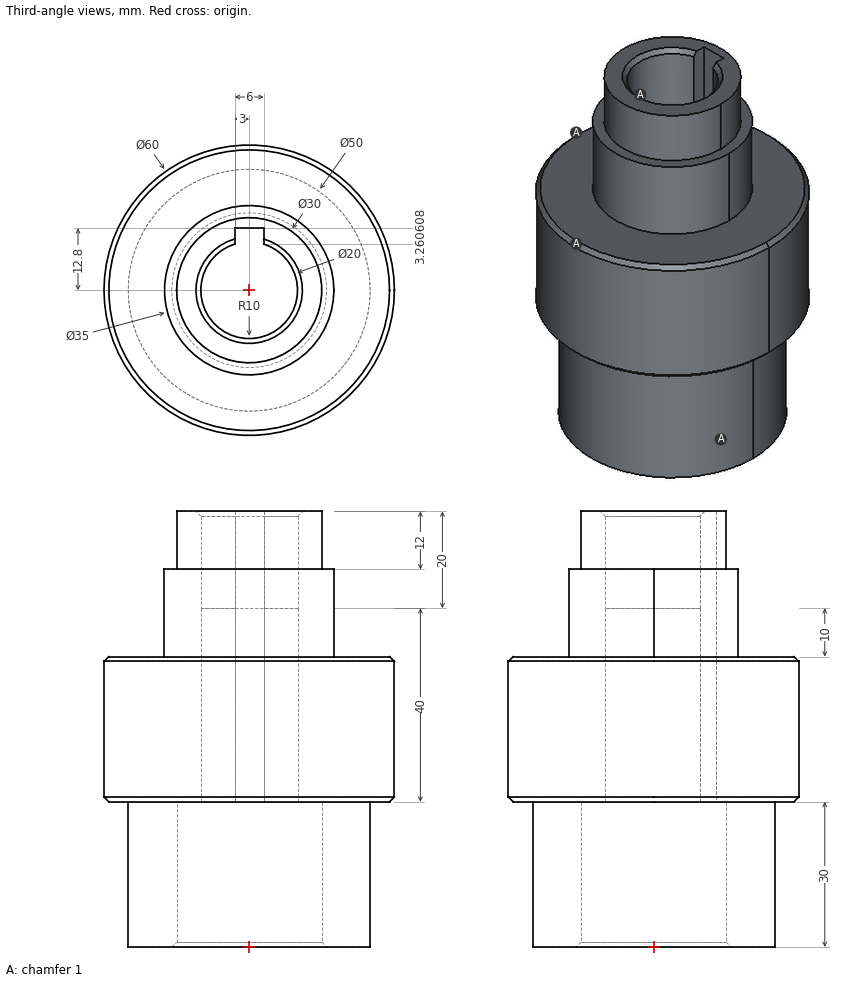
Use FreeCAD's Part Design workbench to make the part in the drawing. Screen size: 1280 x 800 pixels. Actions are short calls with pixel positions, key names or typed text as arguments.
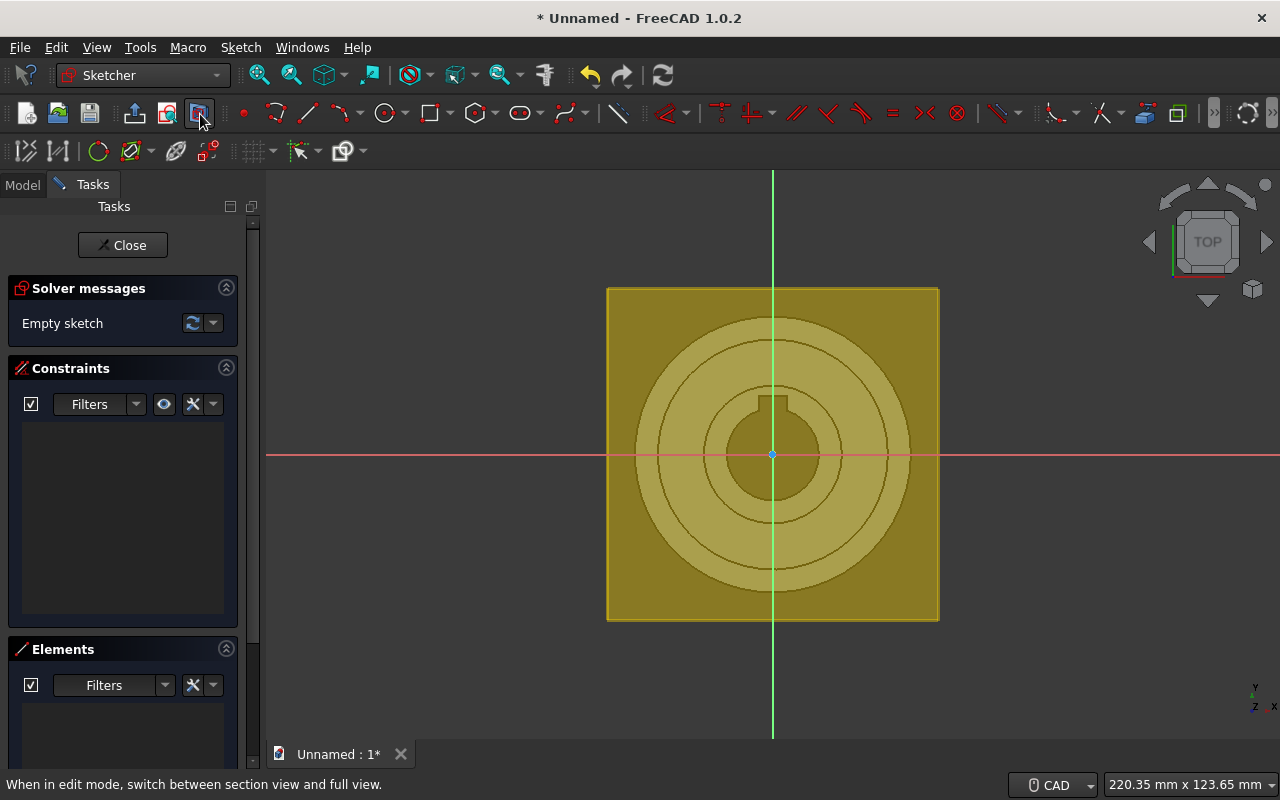
key(g)
key(c)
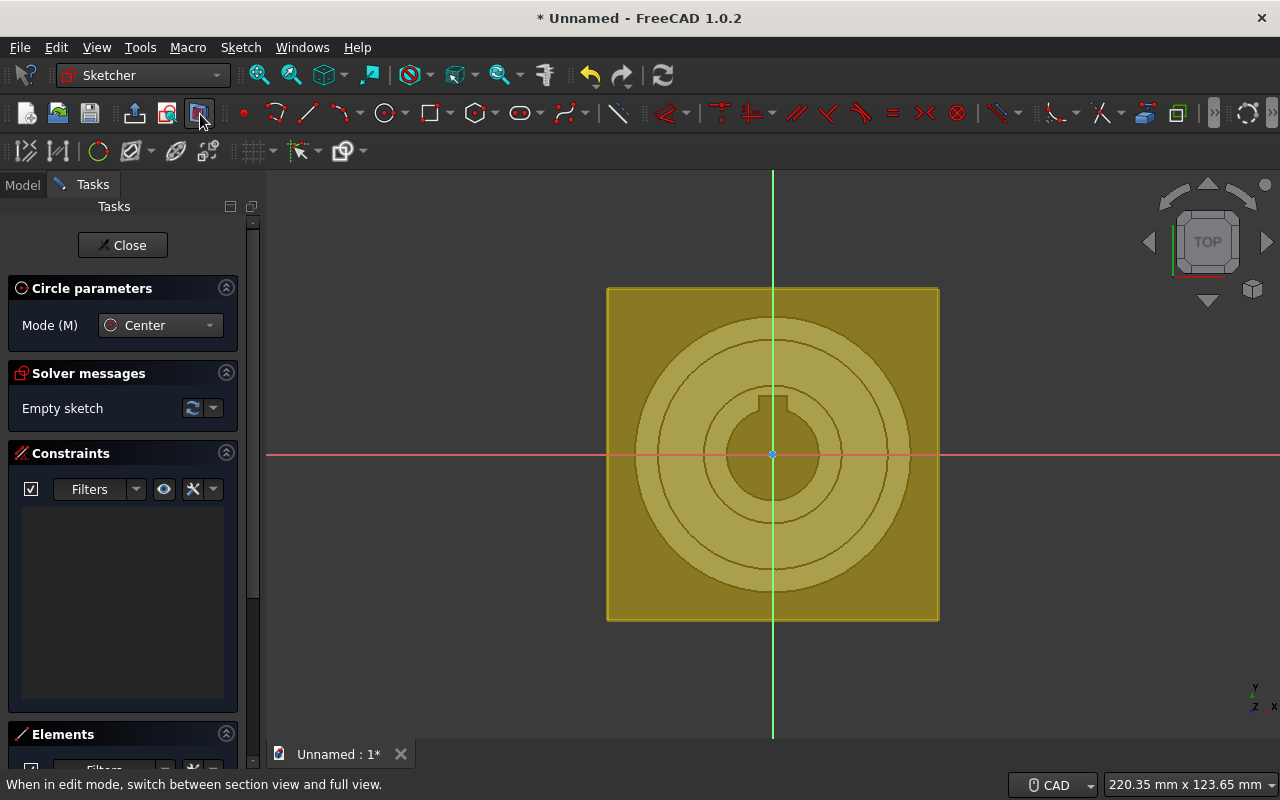
click(773, 454)
move(870, 357)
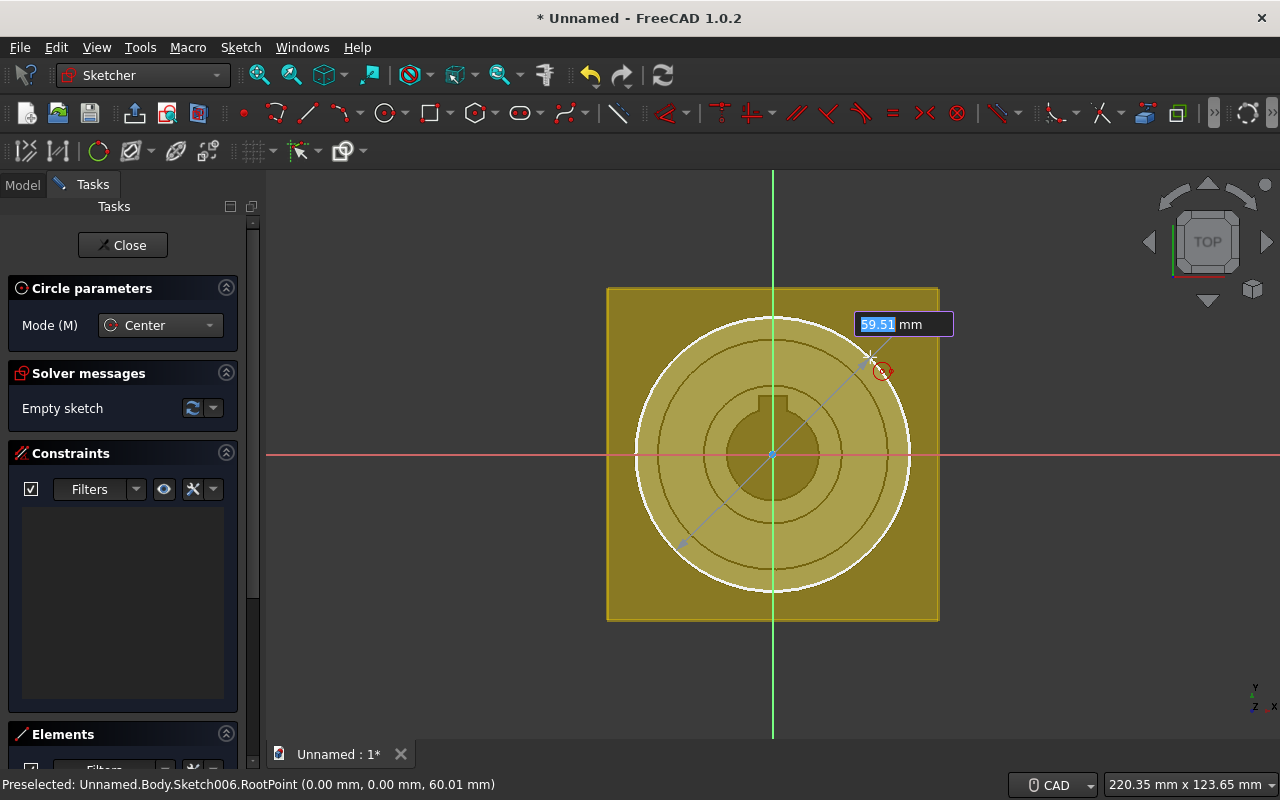
text(60)
key(Return)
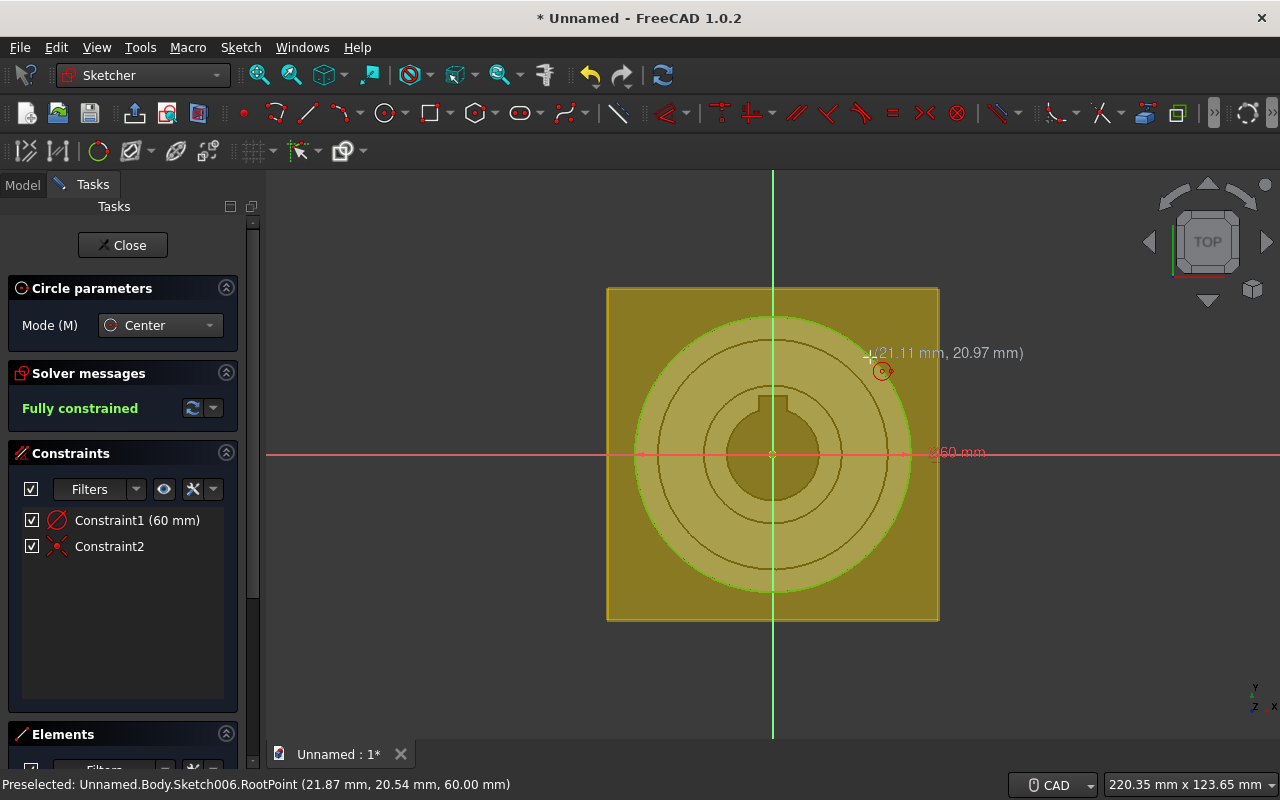
click(773, 454)
move(830, 398)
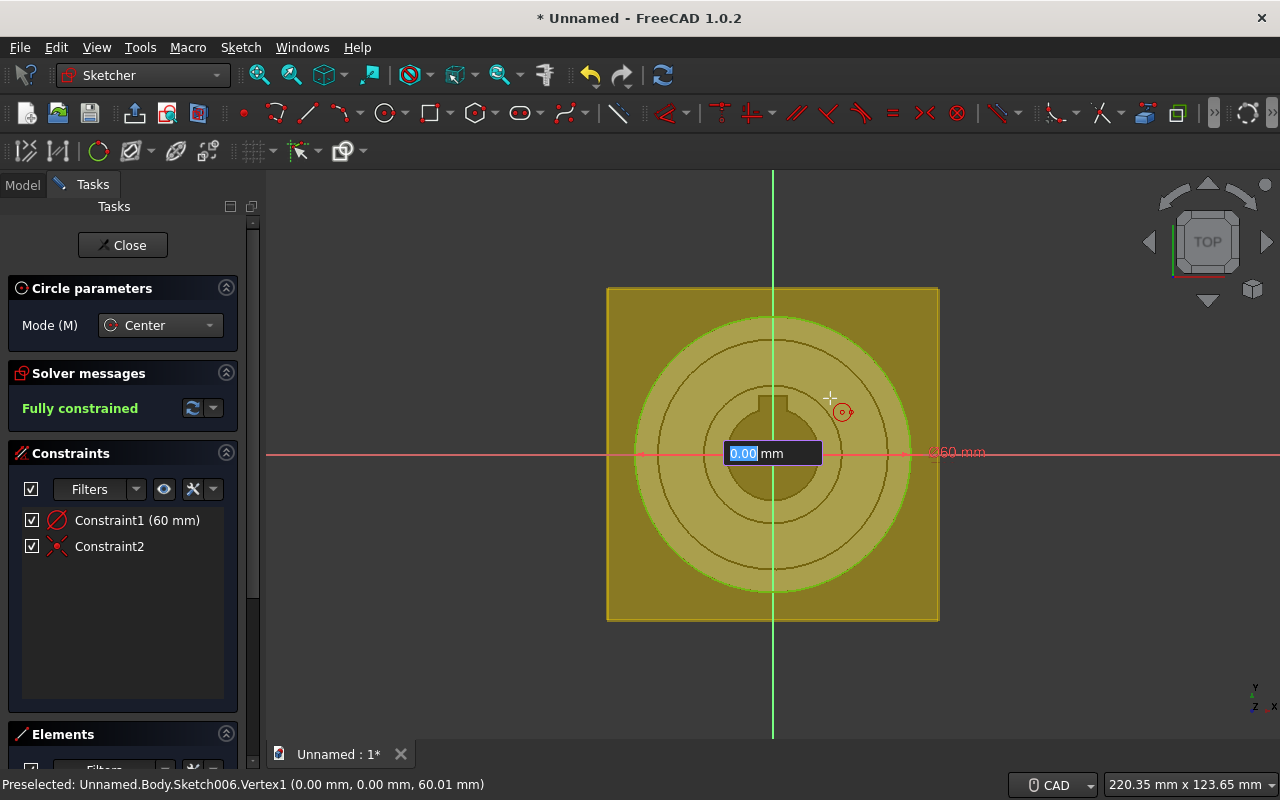
text(35)
key(Return)
key(Escape)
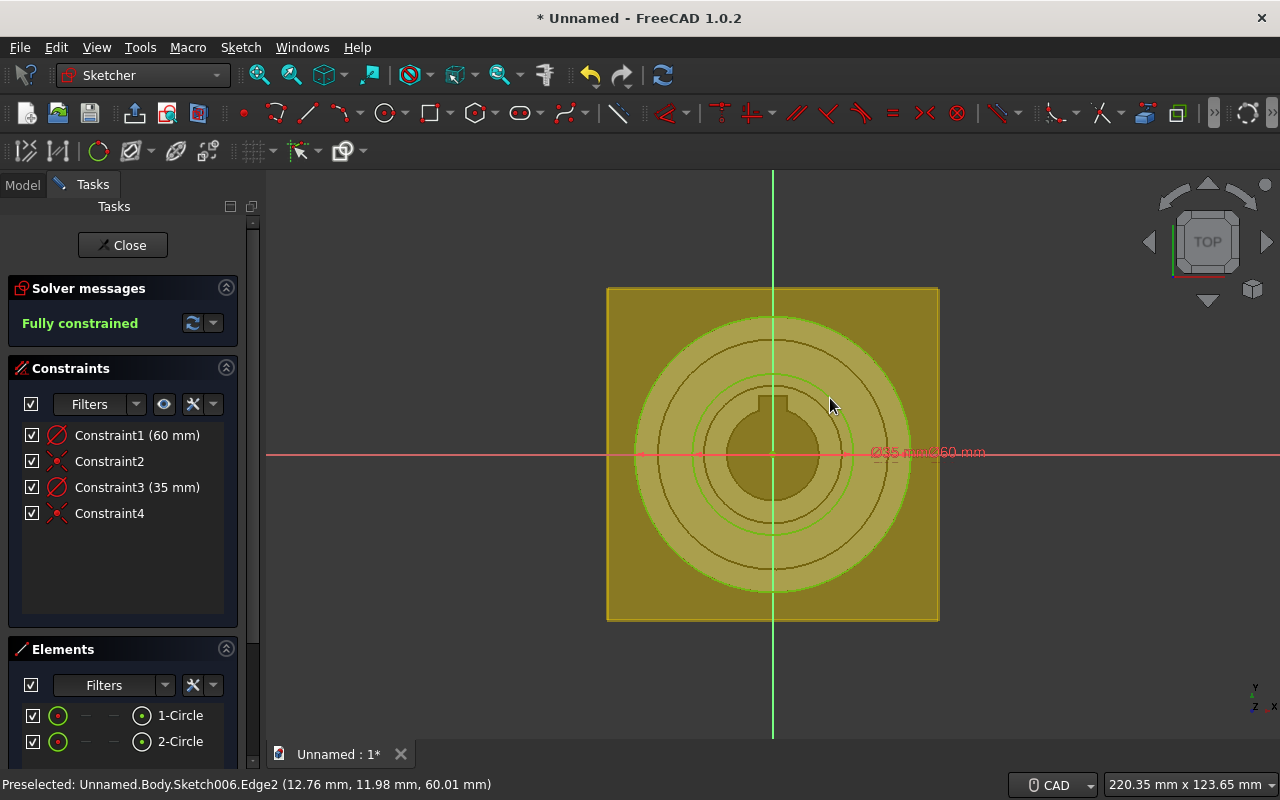
click(123, 245)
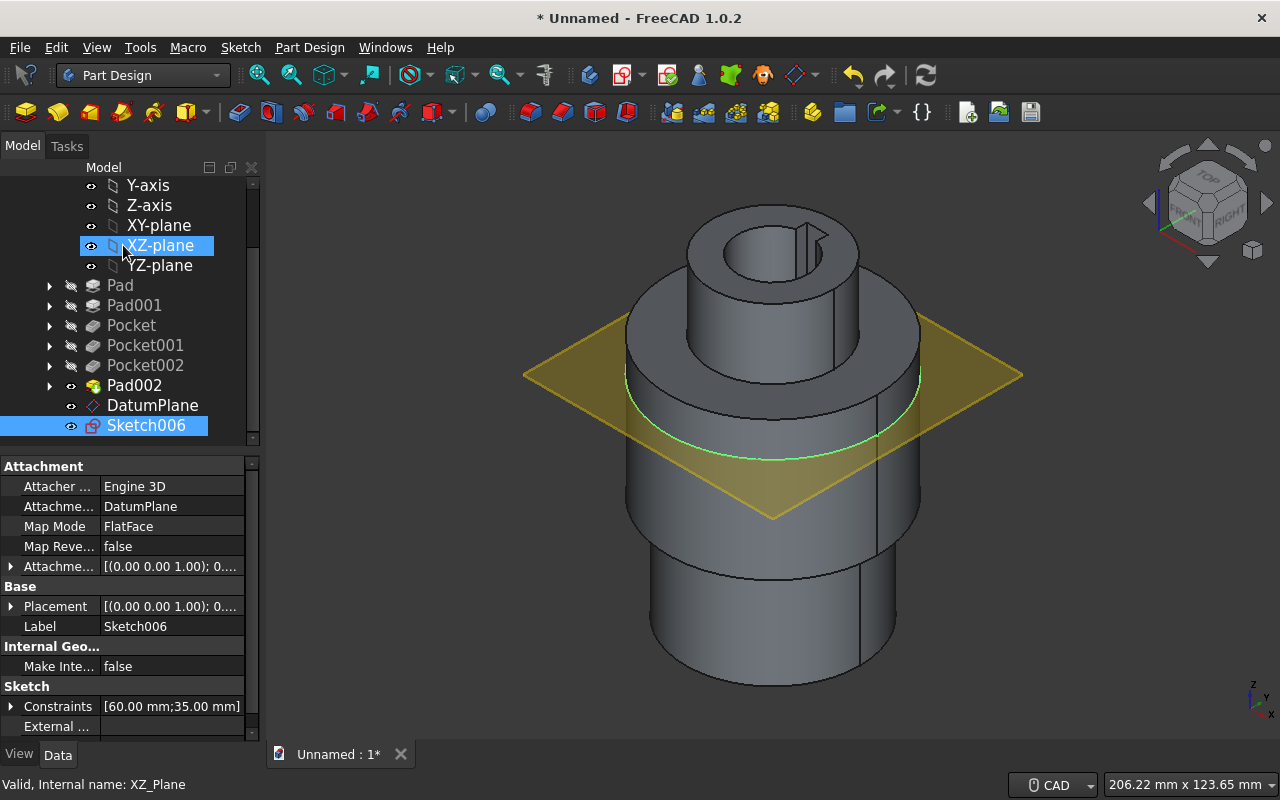
click(240, 112)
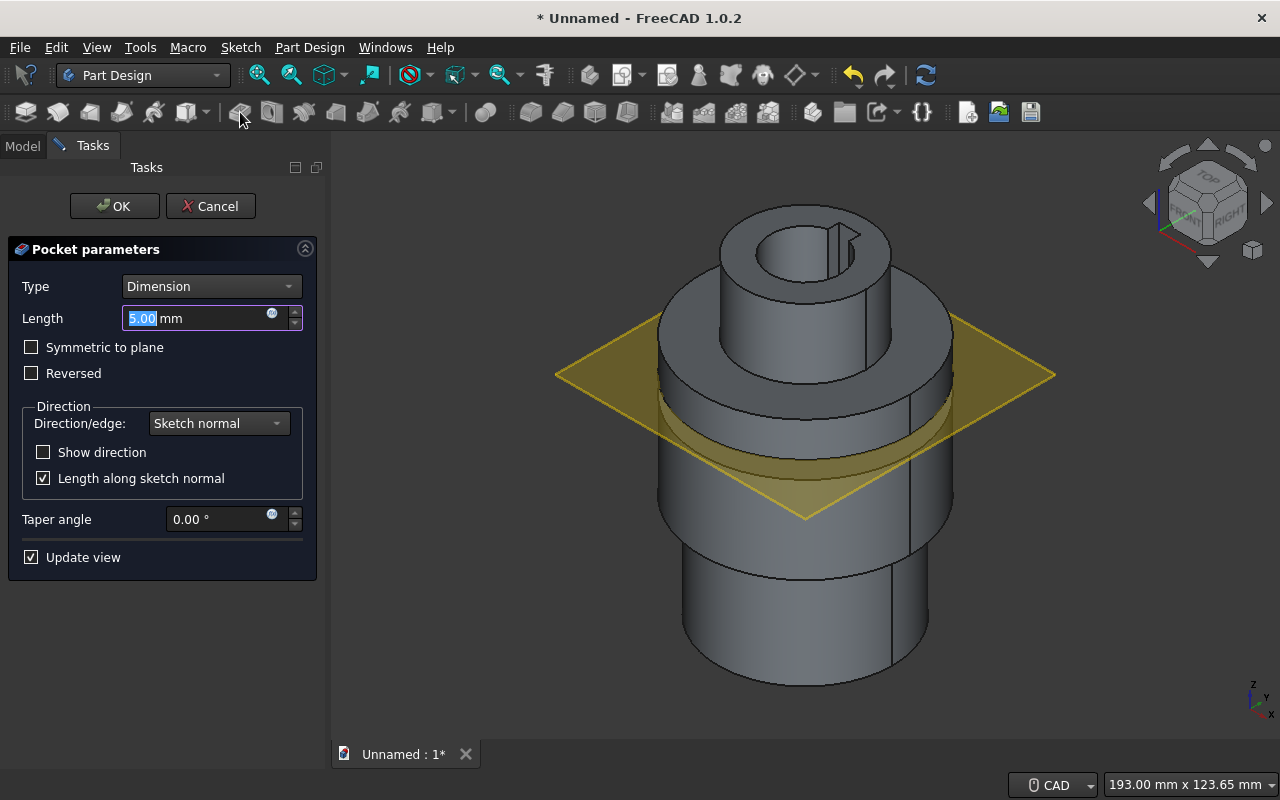
text(10)
key(Tab)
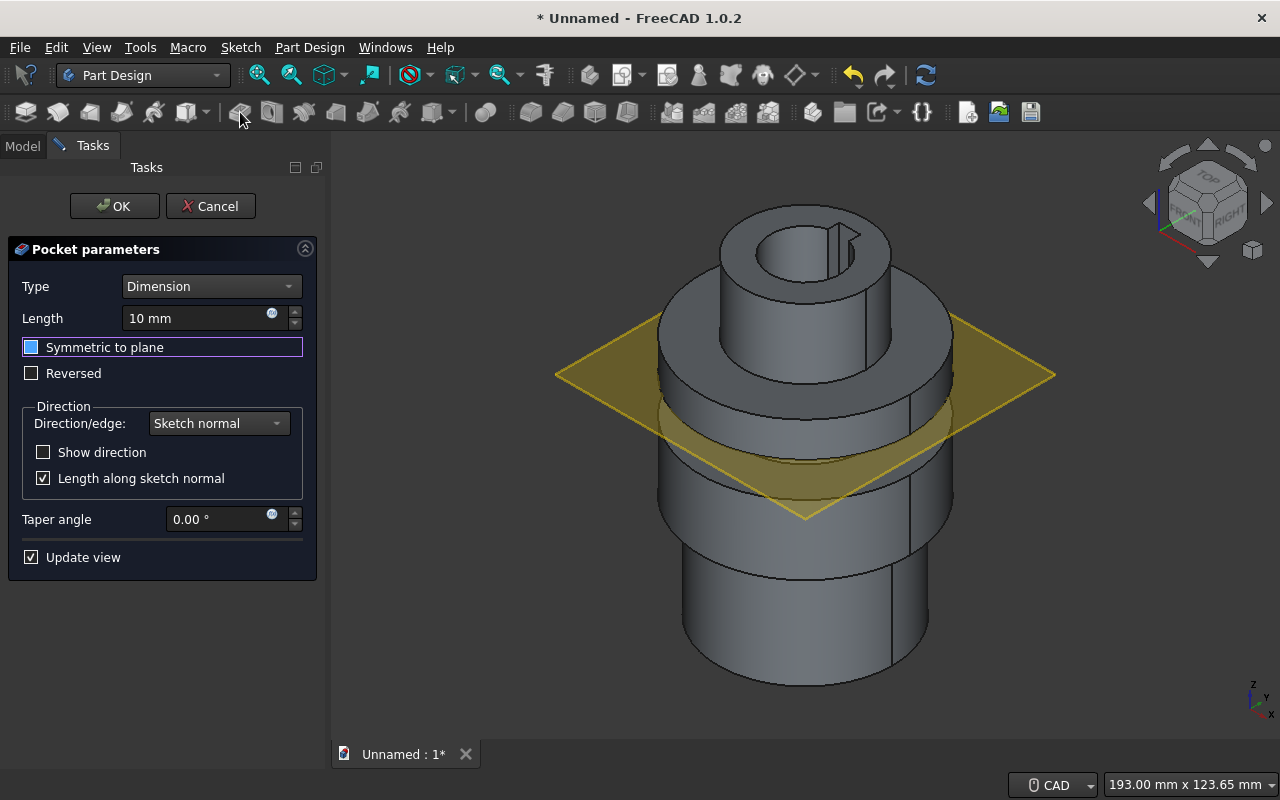
click(30, 373)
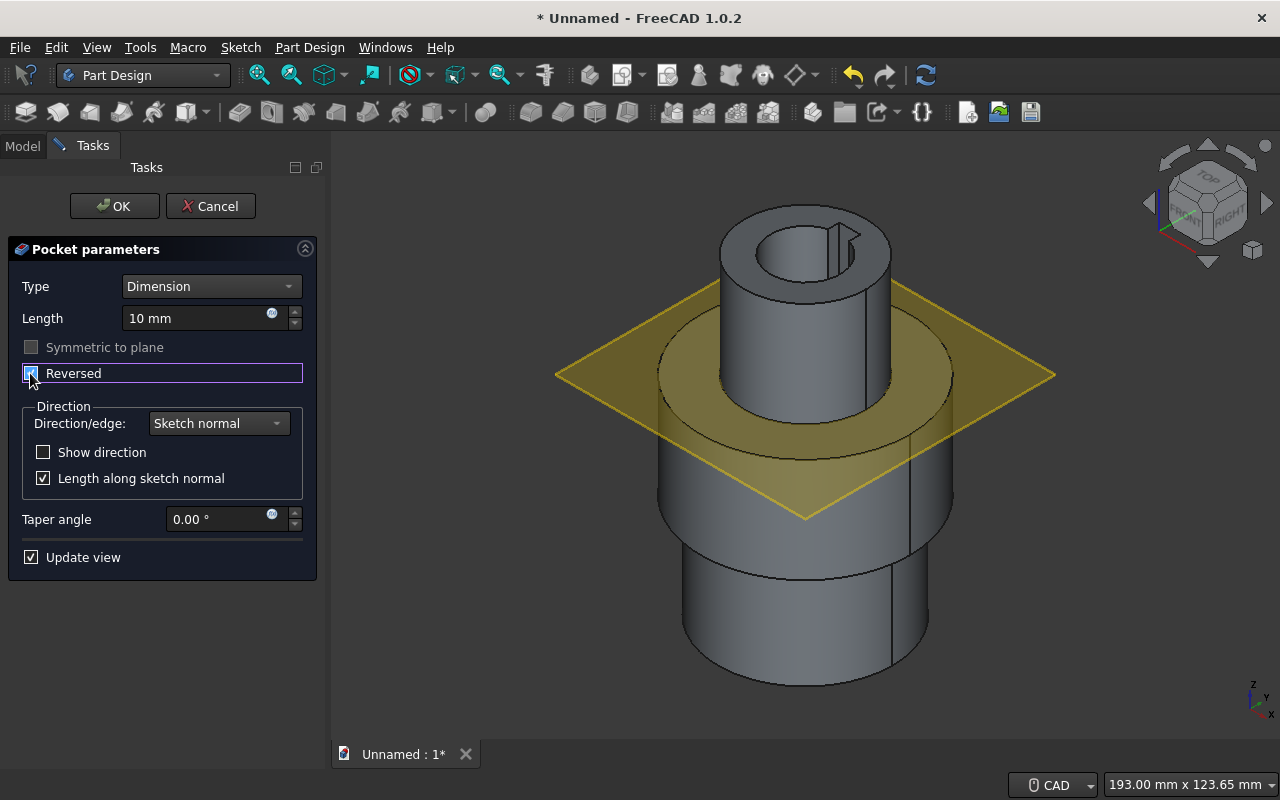
click(115, 206)